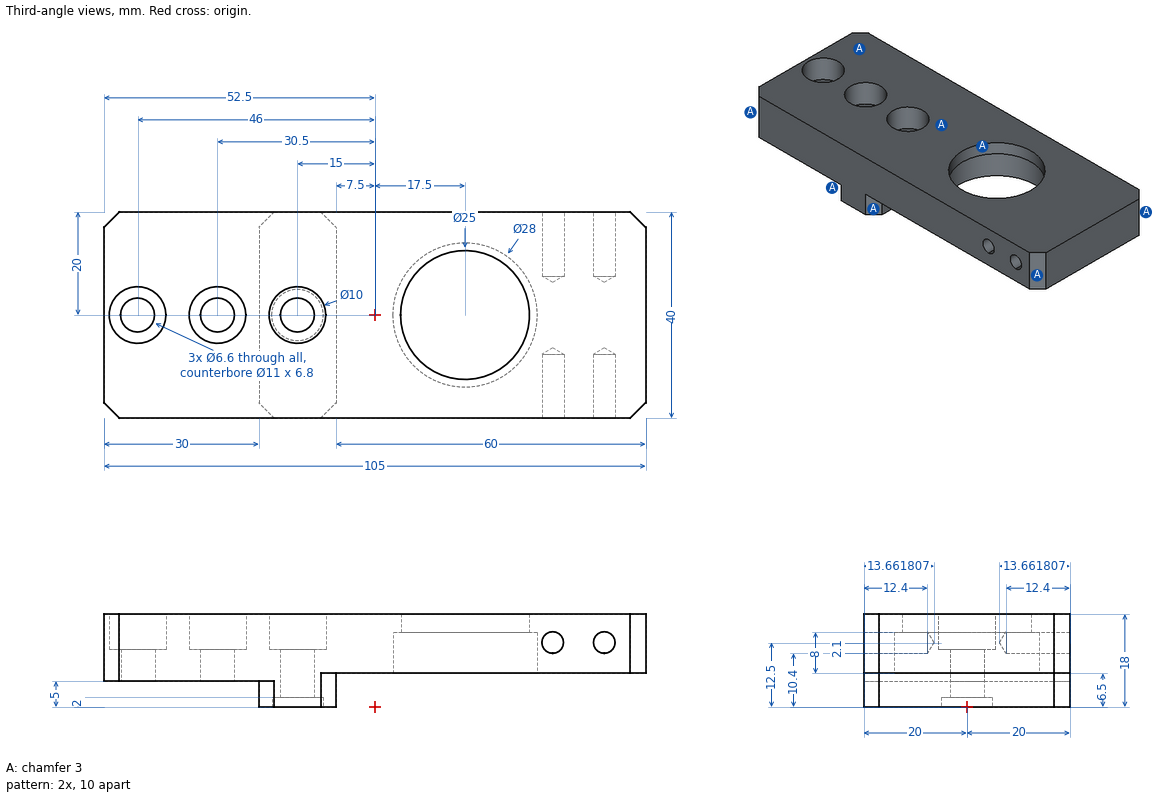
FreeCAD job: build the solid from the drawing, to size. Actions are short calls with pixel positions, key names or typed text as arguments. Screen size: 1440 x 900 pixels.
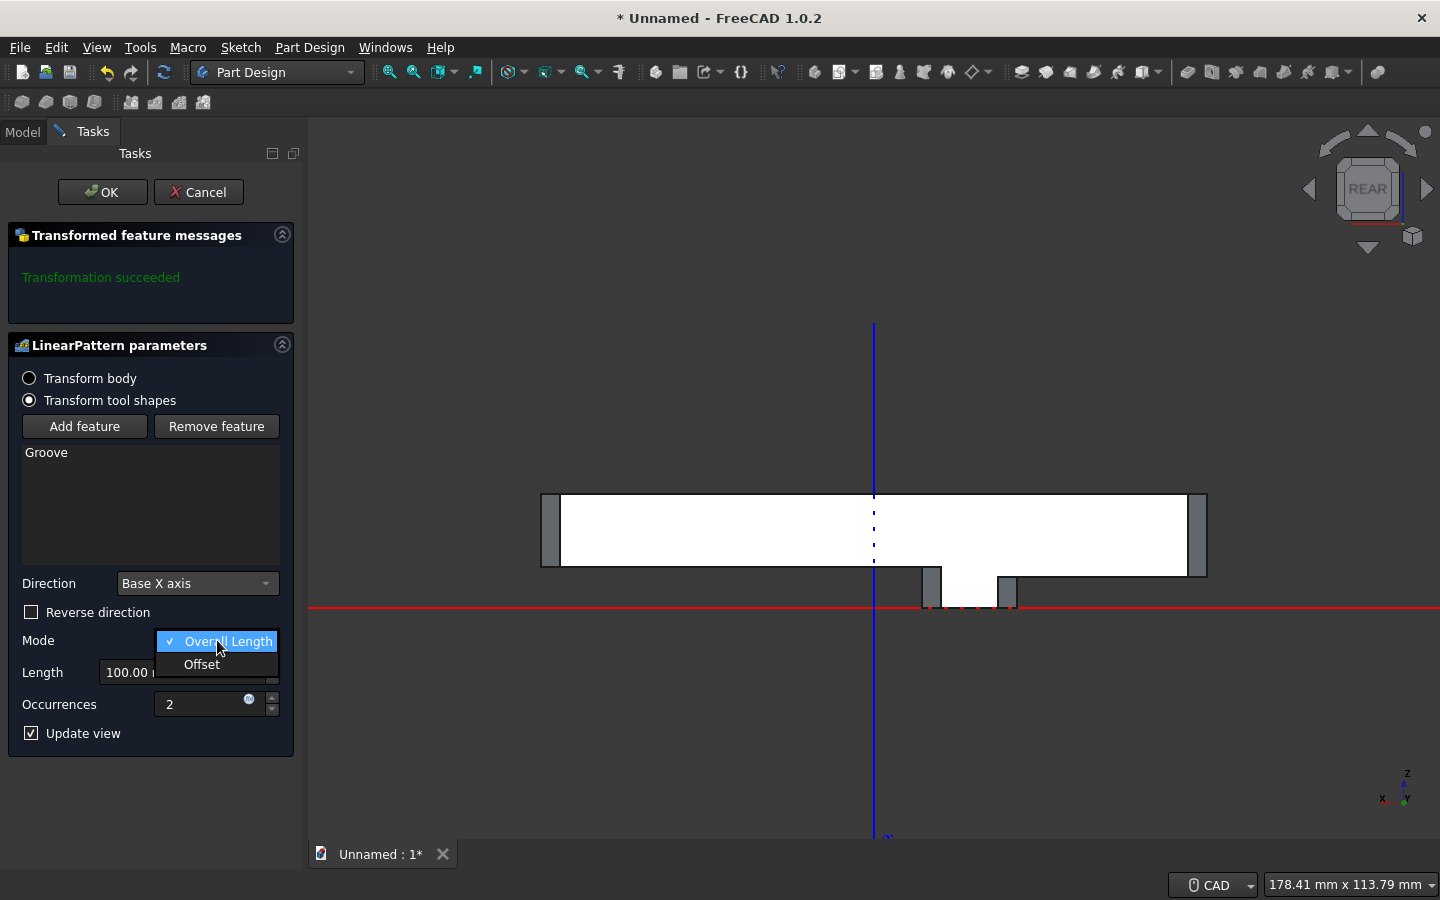
click(216, 664)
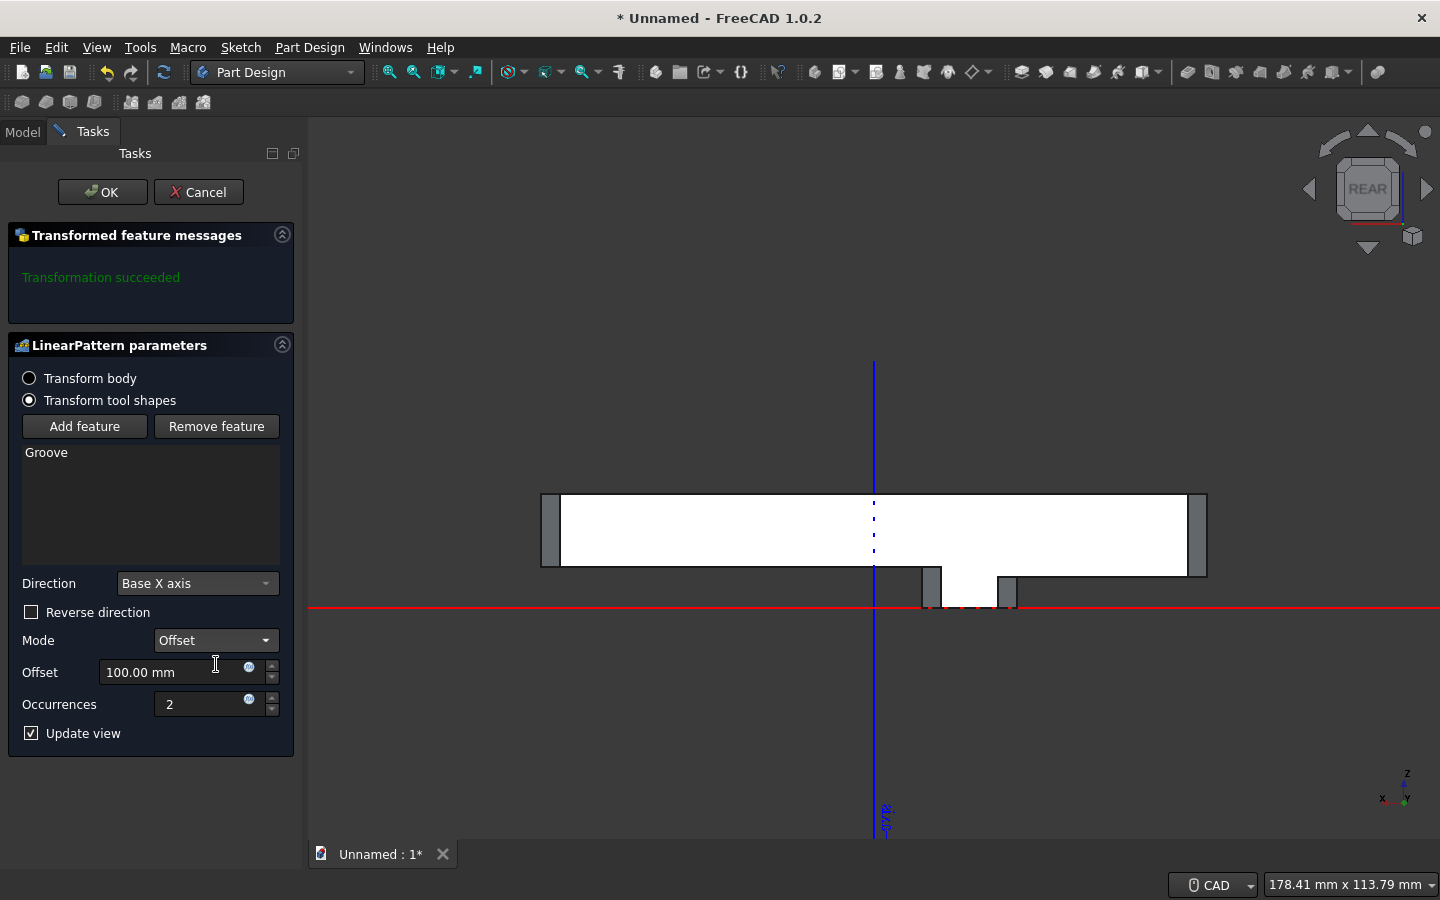
triple_click(182, 672)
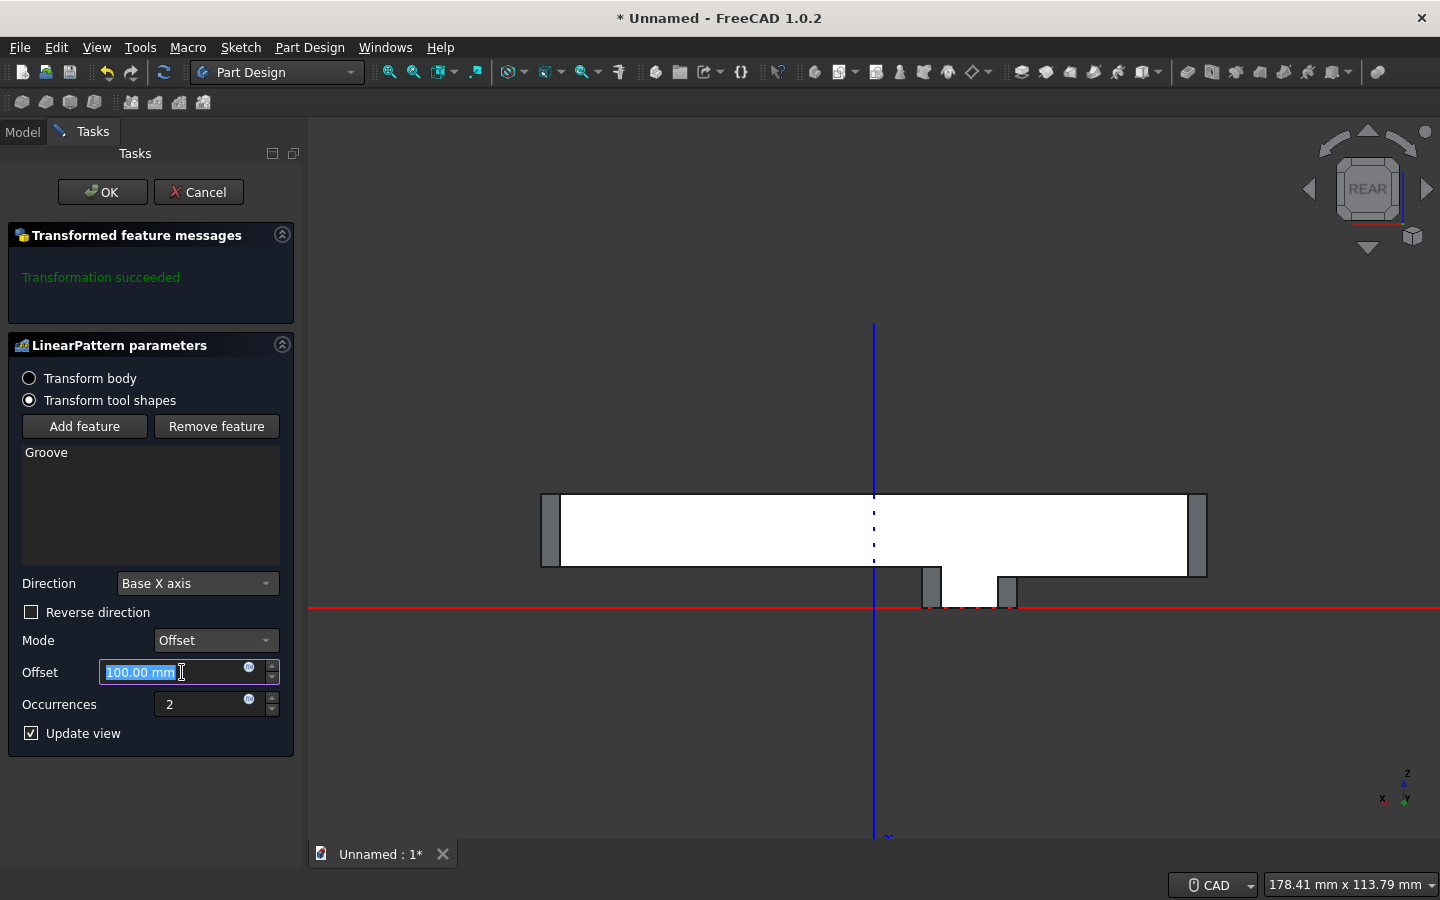
text(10)
key(Tab)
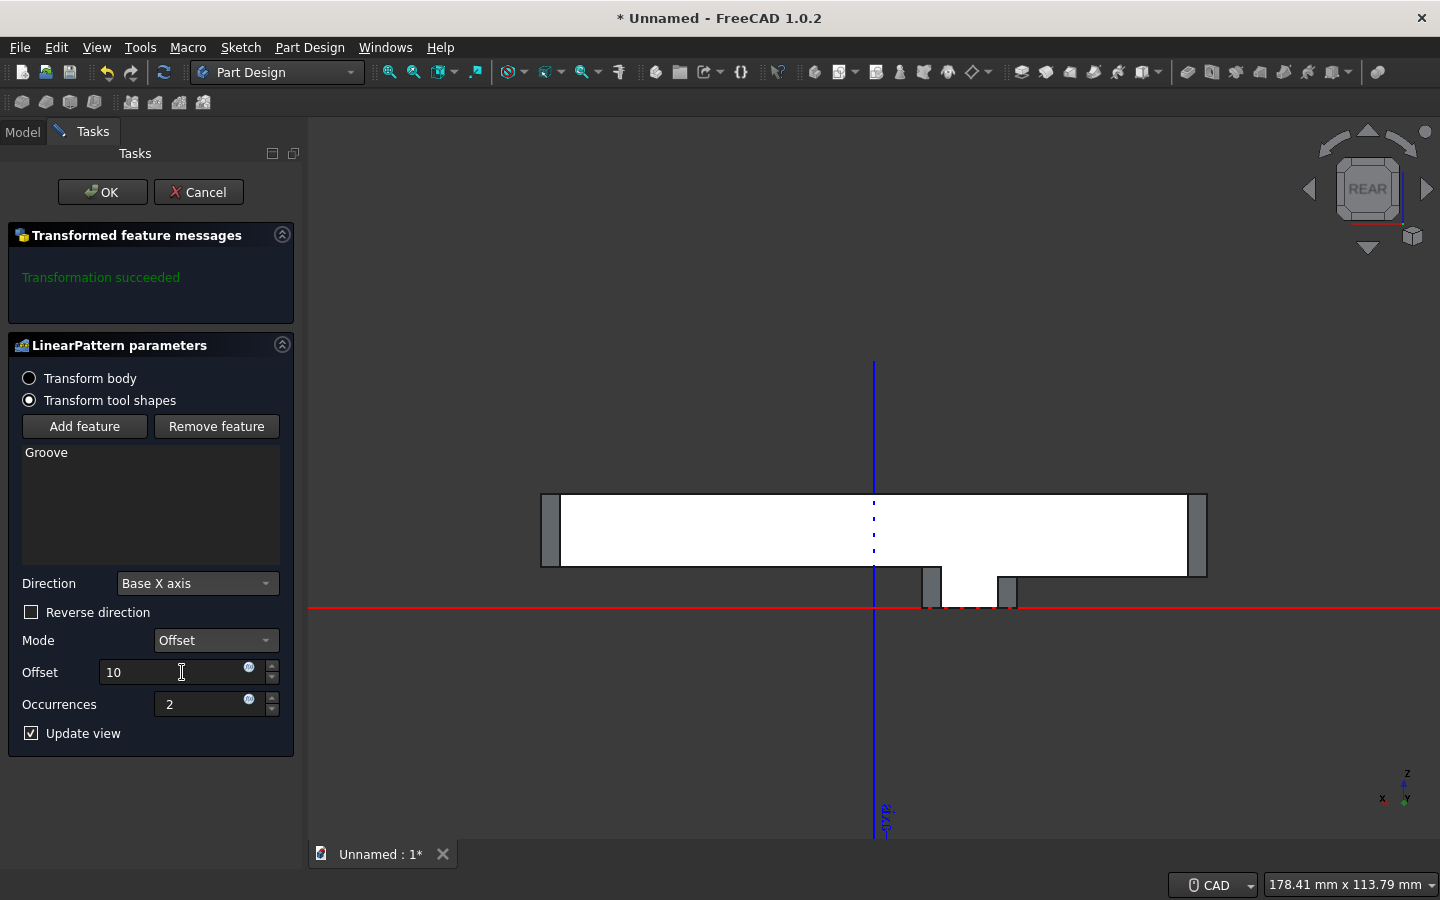
triple_click(209, 704)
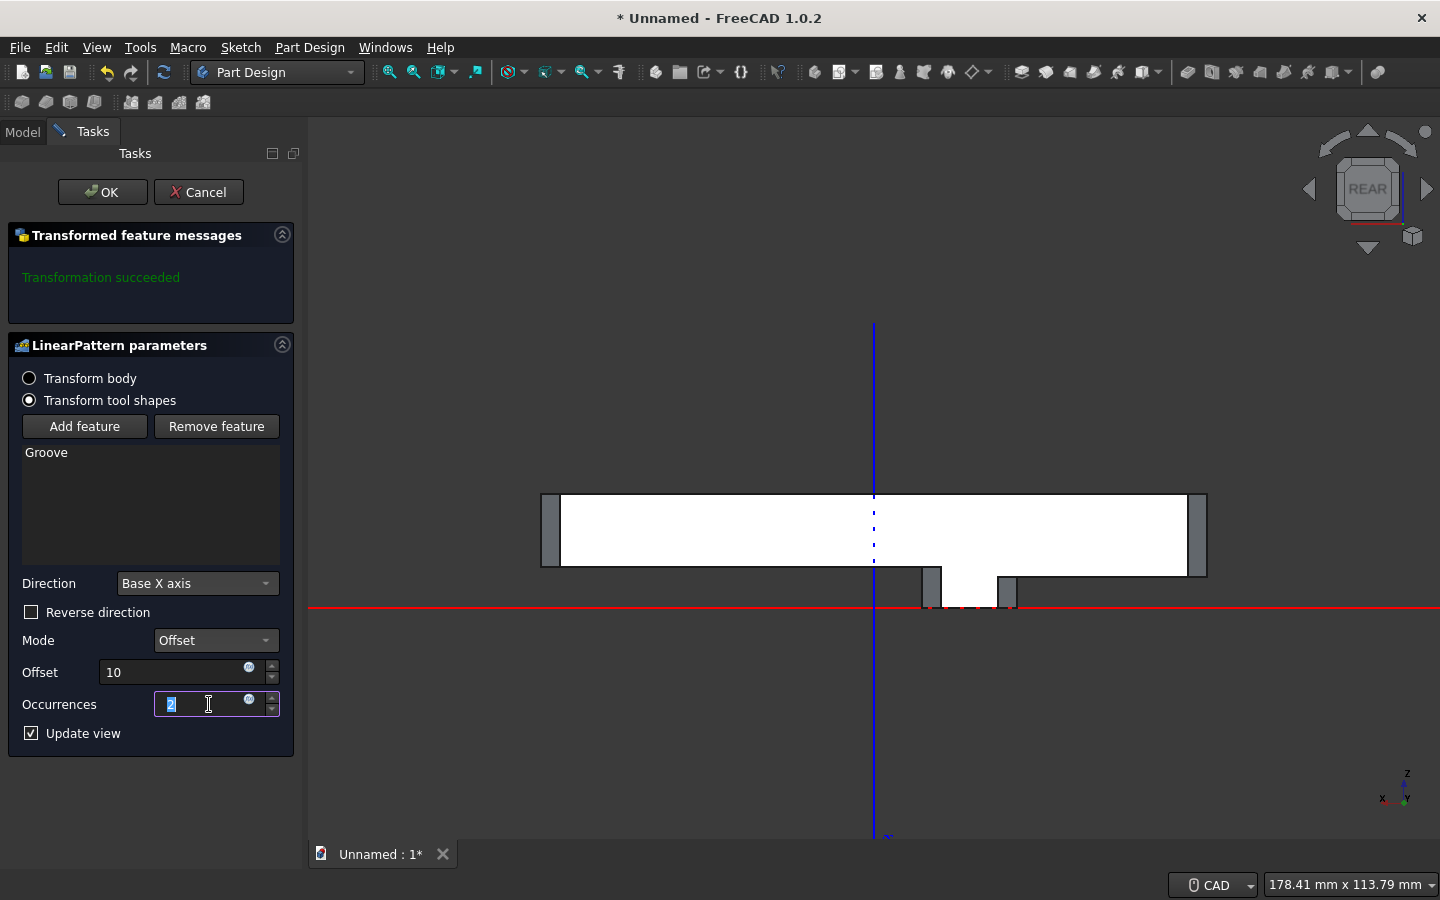
text(2)
key(Tab)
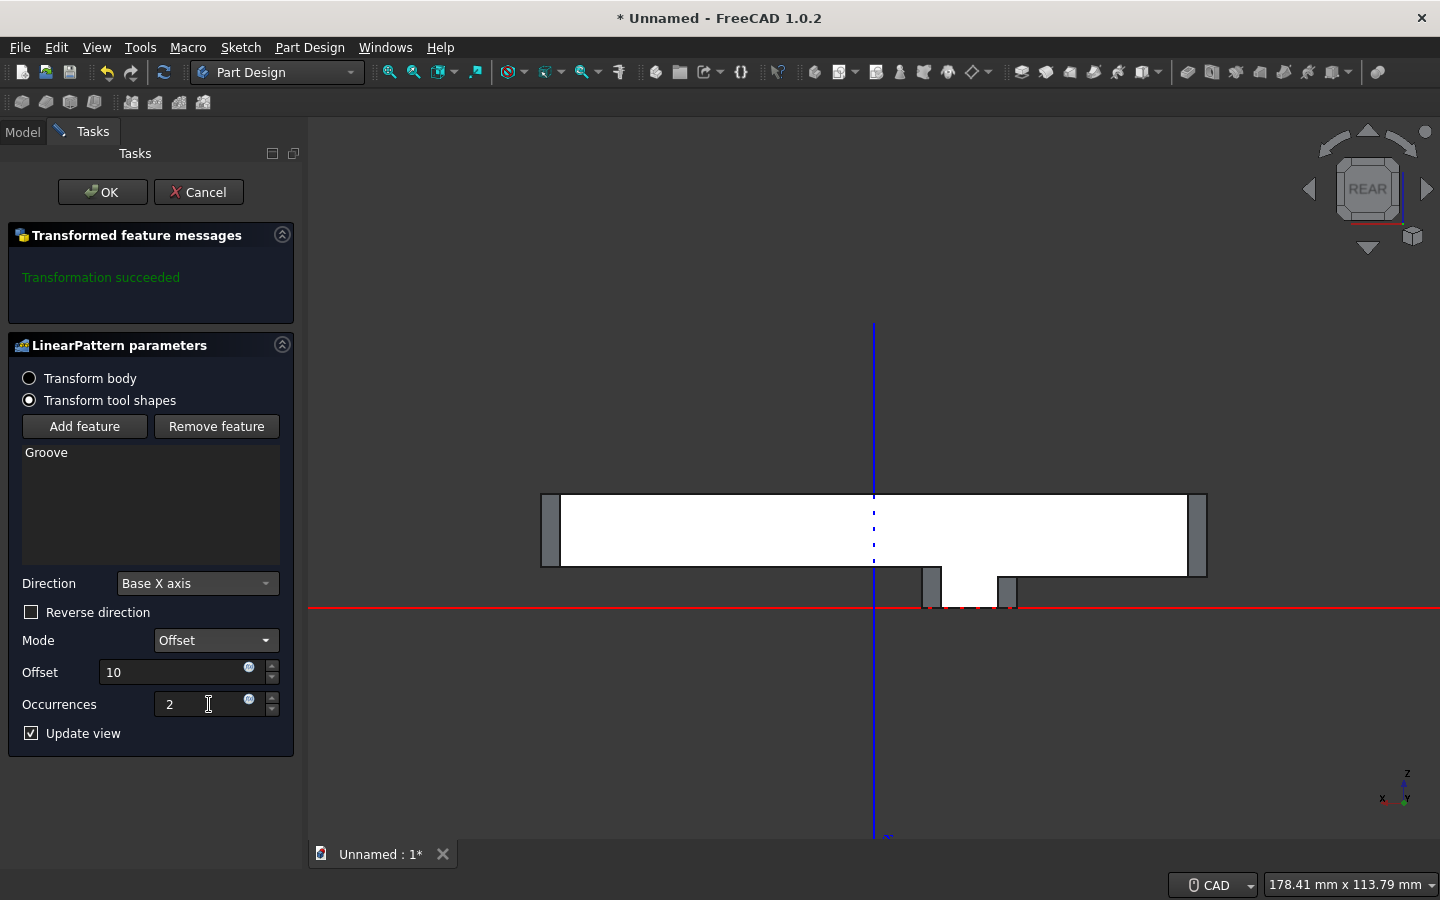
click(30, 612)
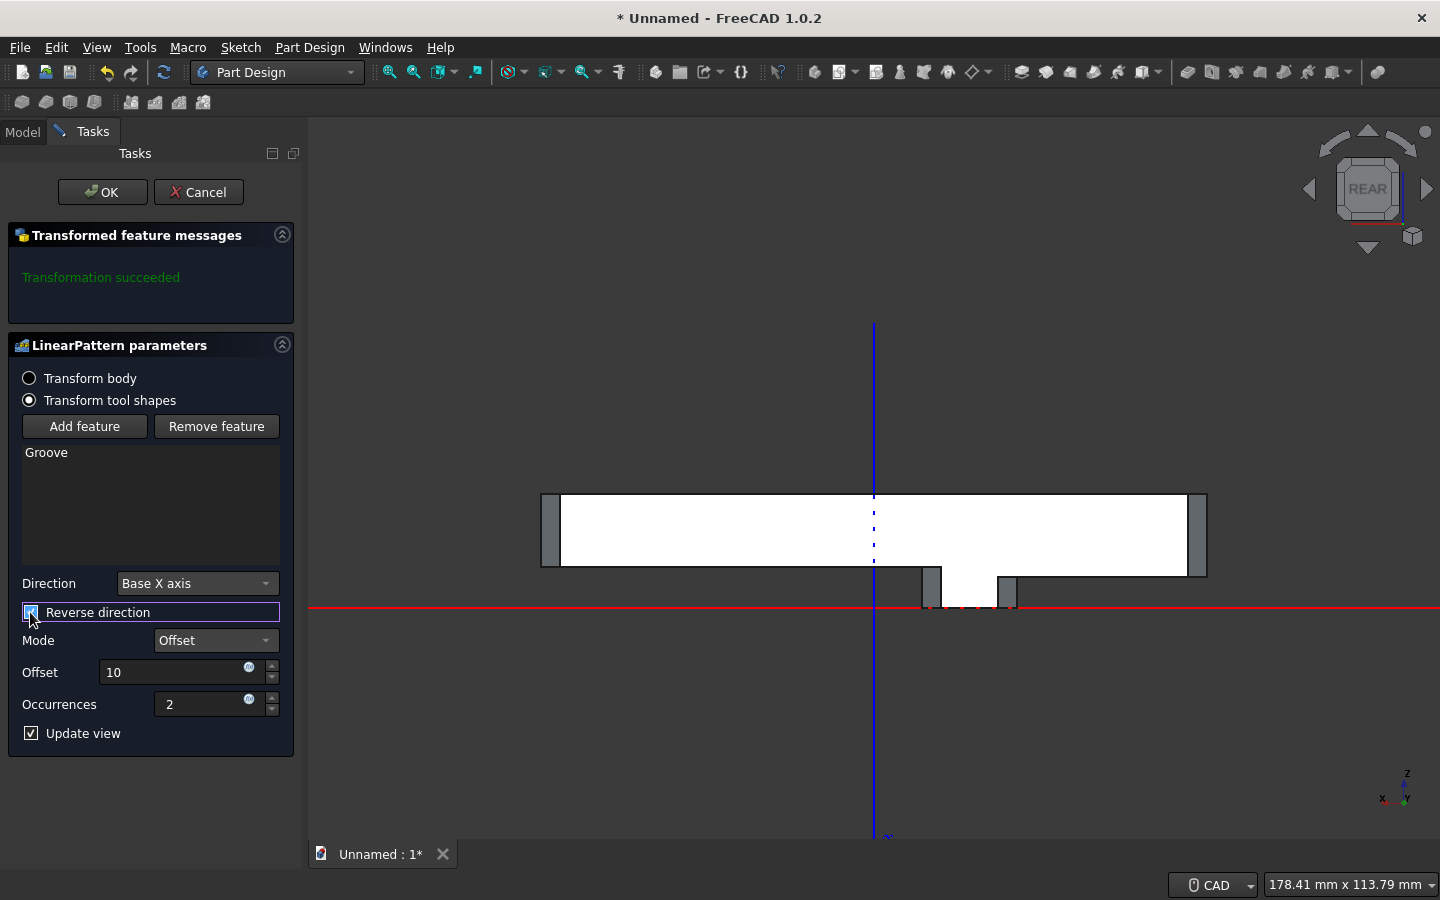
click(103, 192)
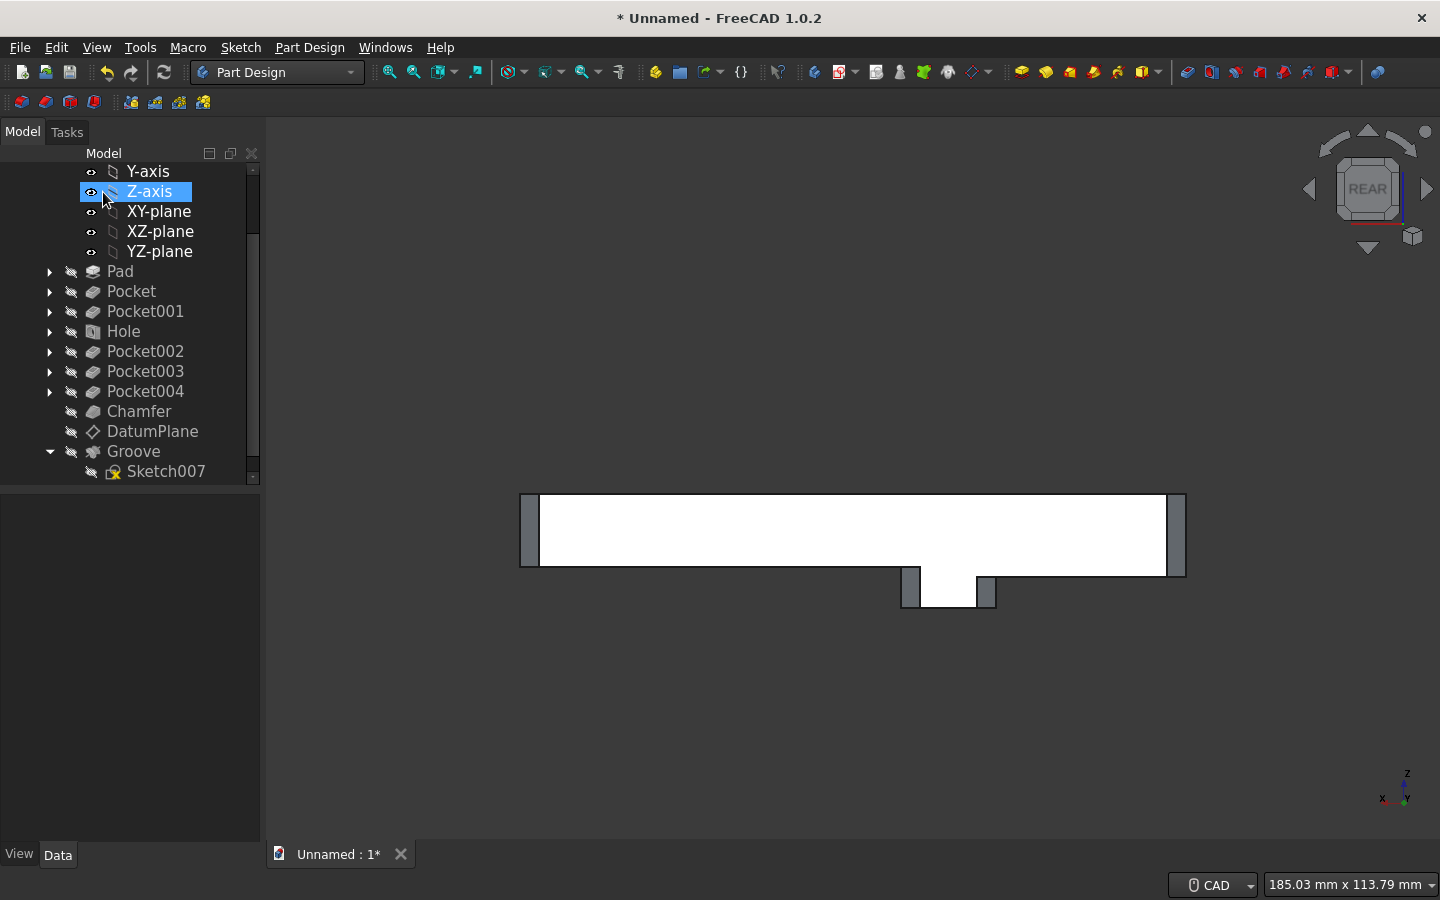
click(116, 452)